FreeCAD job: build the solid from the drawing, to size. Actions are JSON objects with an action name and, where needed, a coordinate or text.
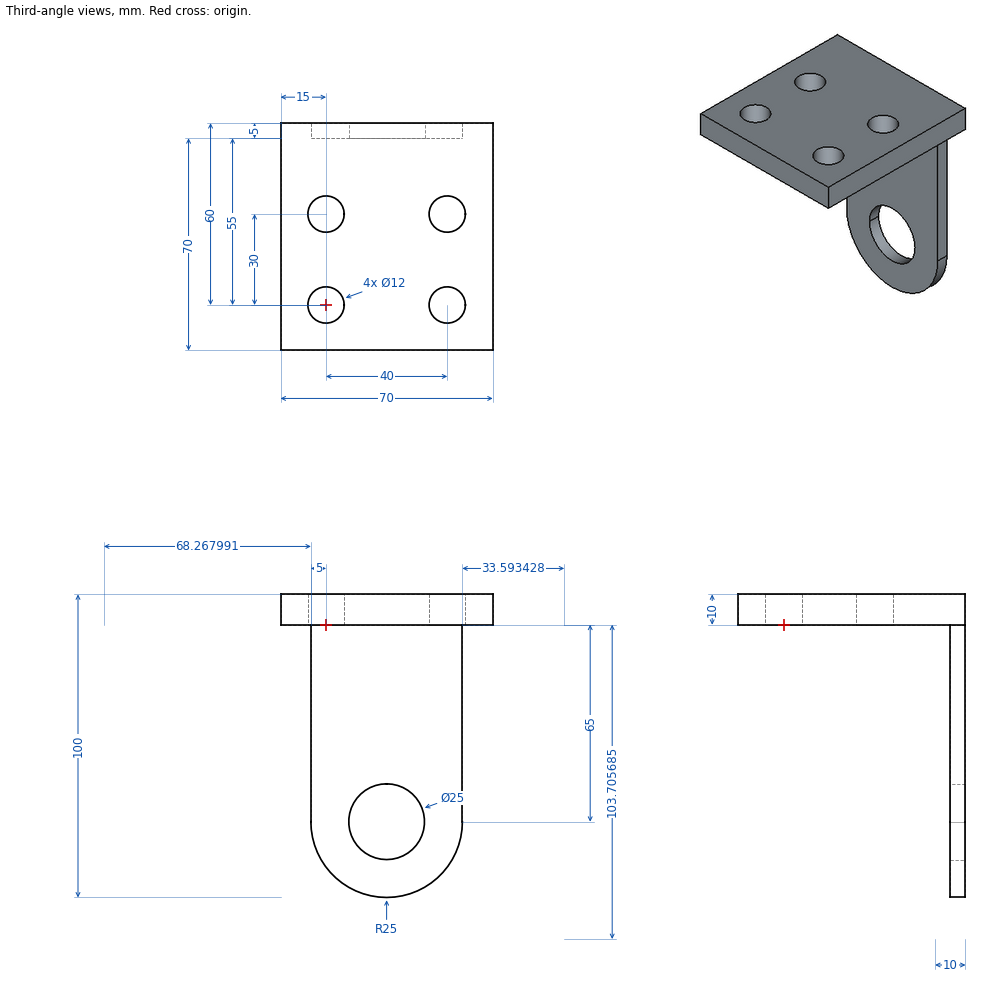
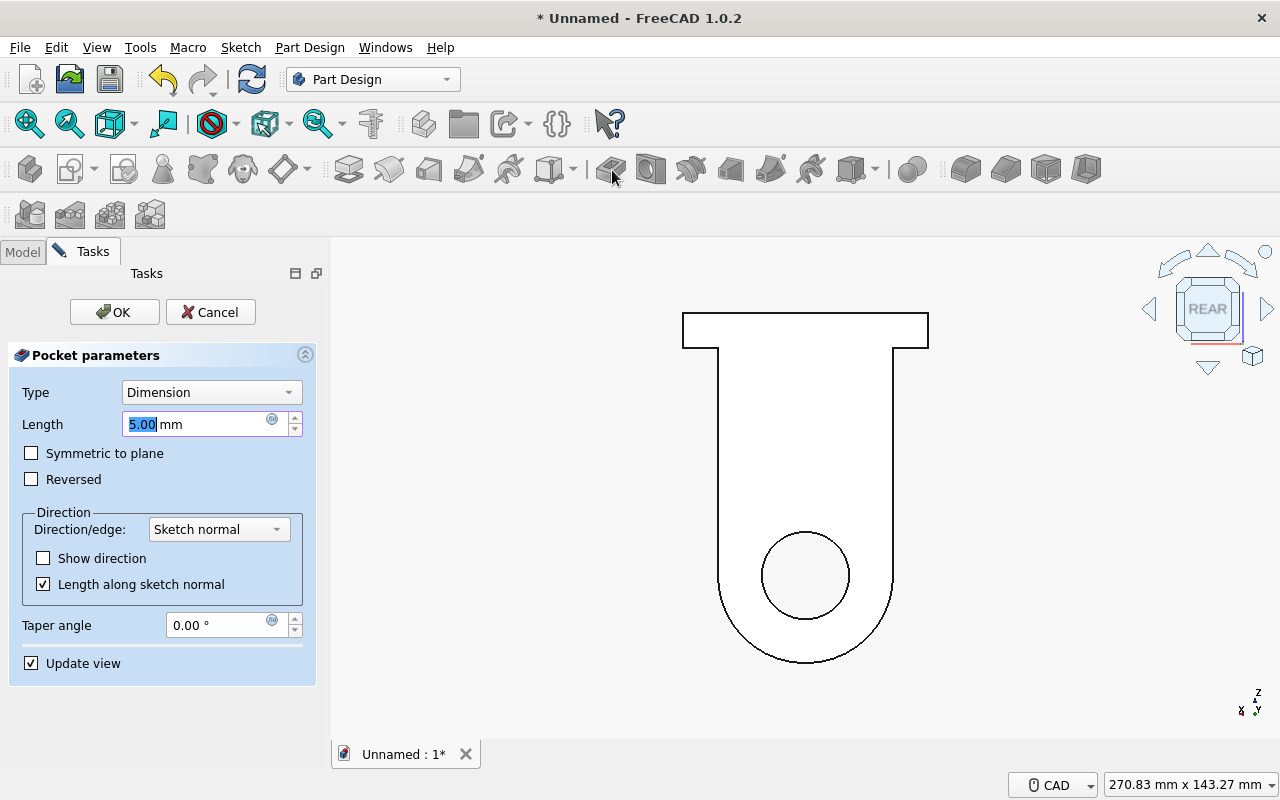
{"action": "type", "text": "10"}
{"action": "key", "text": "Tab"}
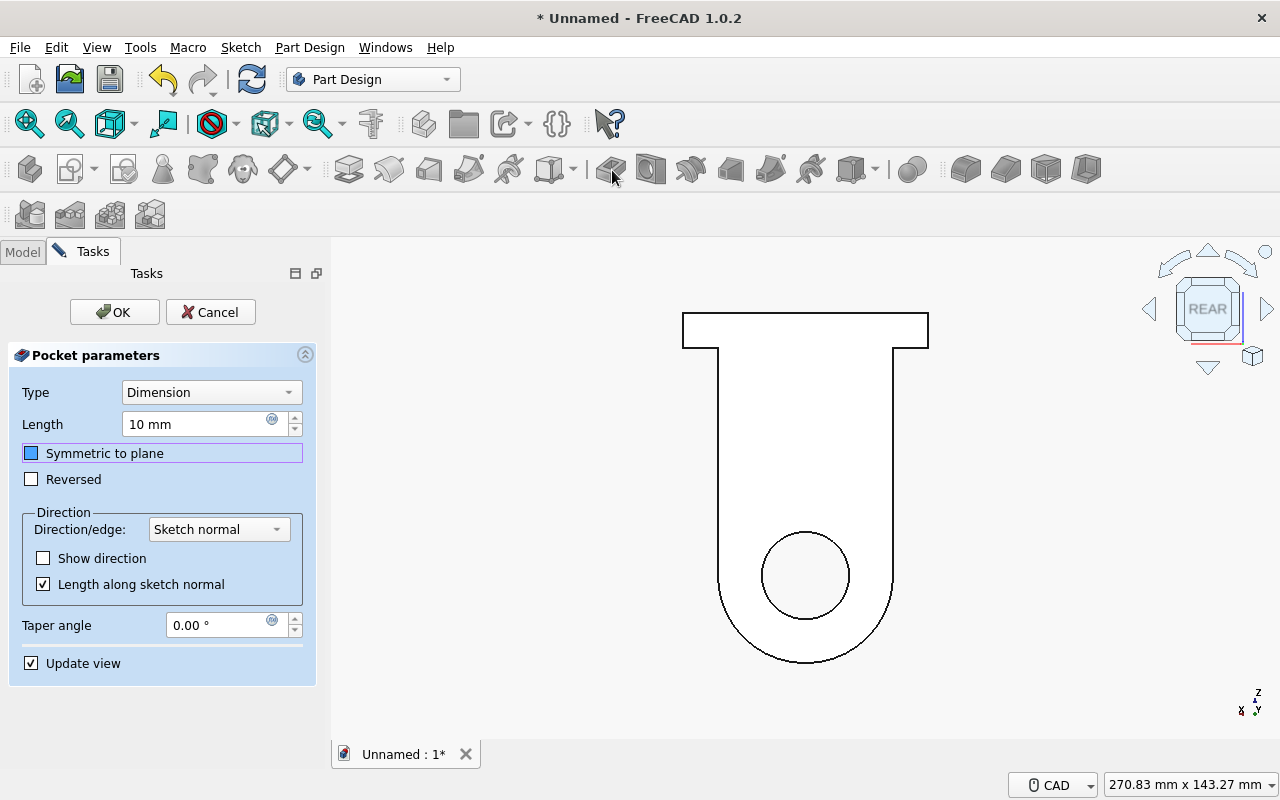
{"action": "left_click", "coordinate": [115, 312]}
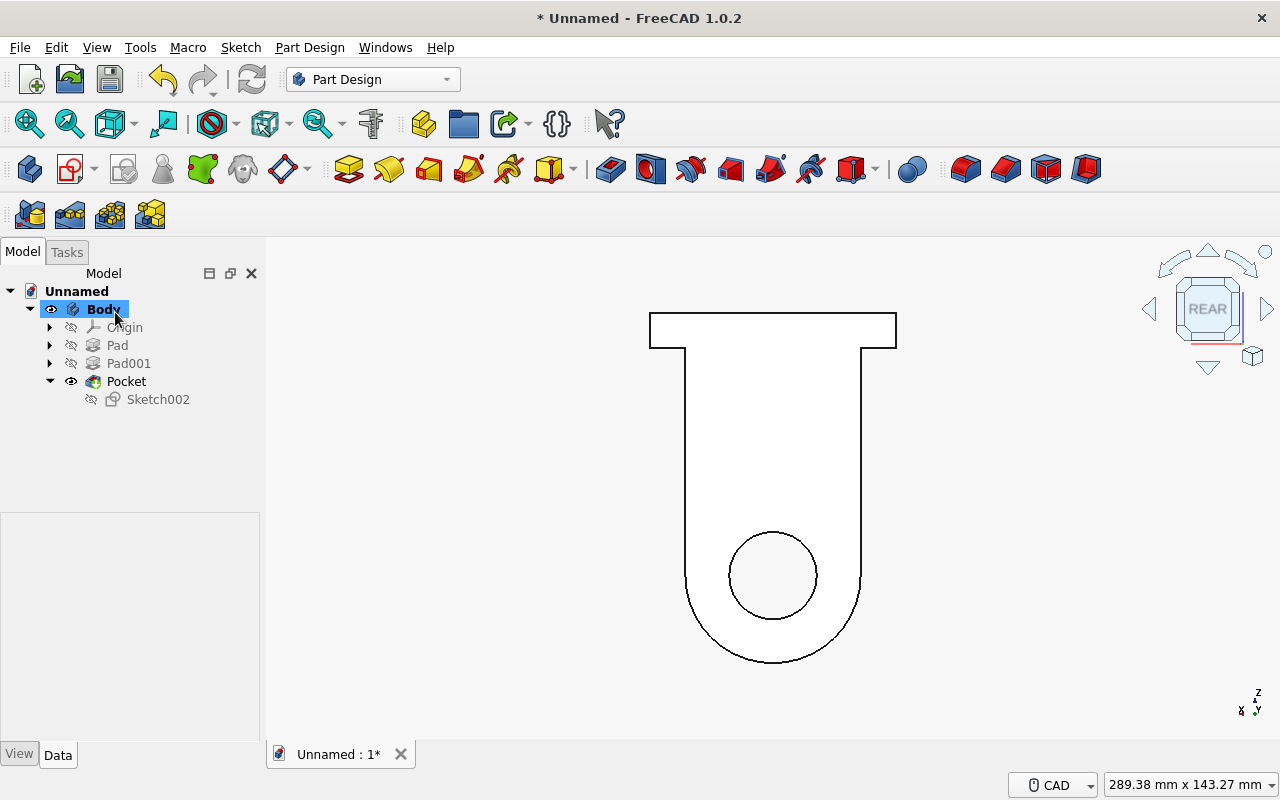
{"action": "key", "text": "0"}